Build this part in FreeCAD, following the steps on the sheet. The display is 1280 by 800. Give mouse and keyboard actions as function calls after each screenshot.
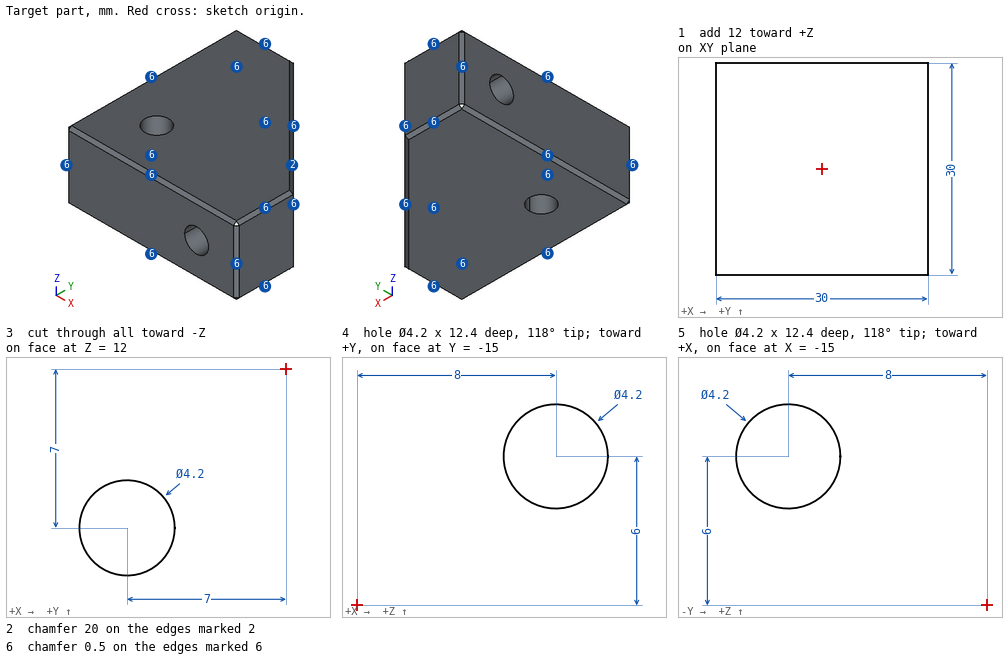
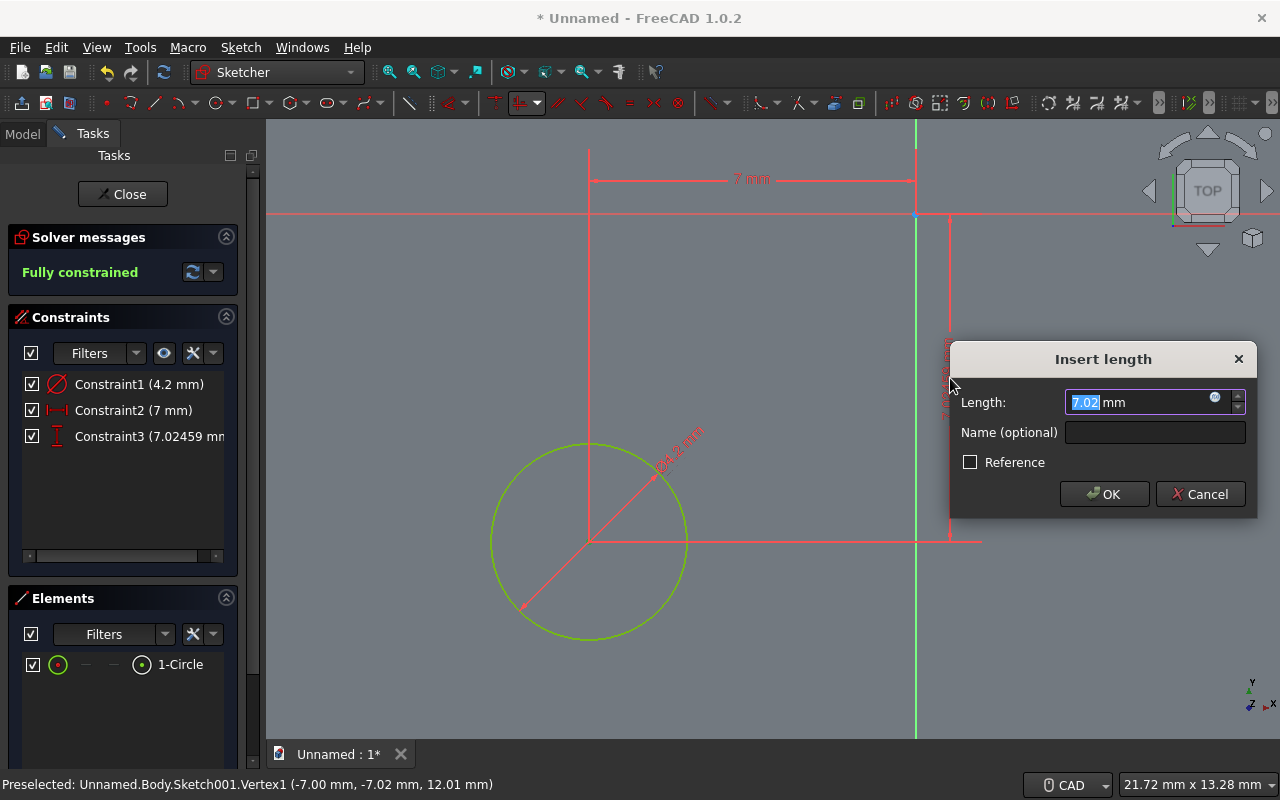
text(7)
key(Return)
key(Escape)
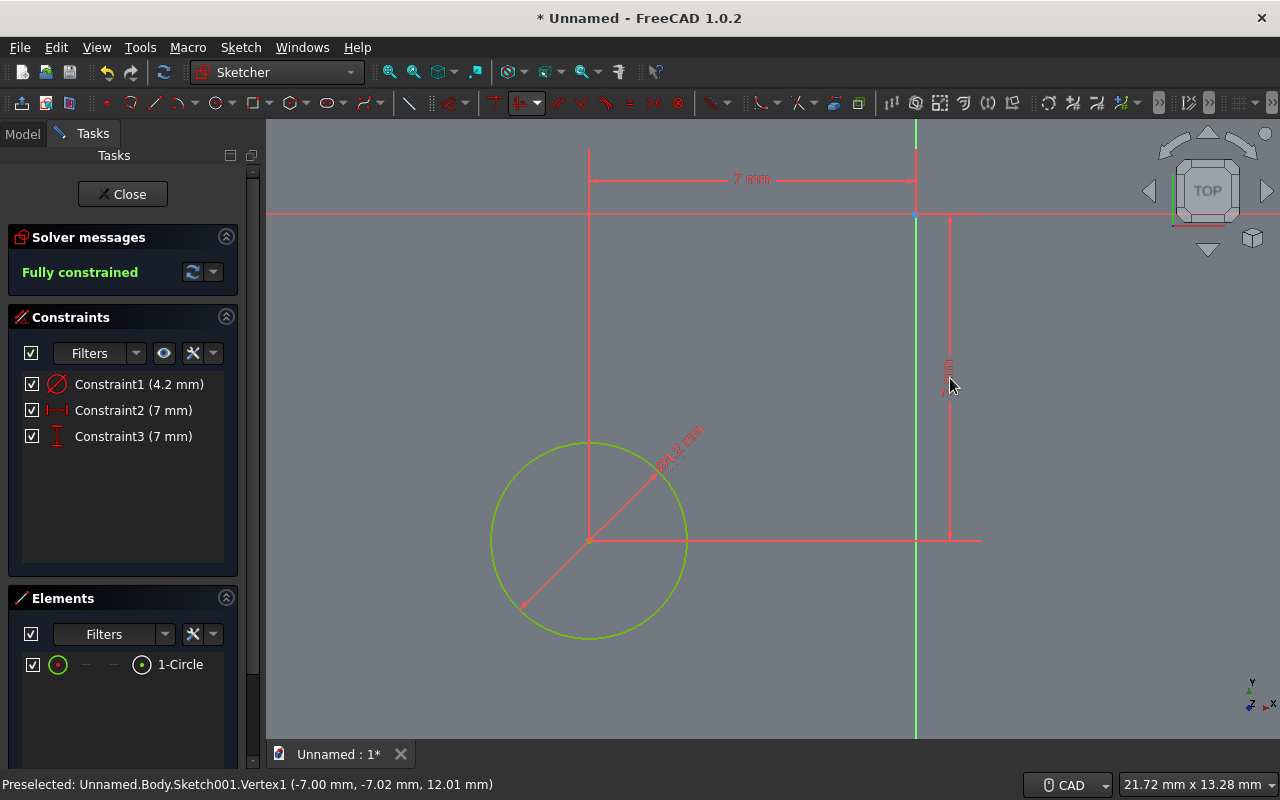
click(123, 194)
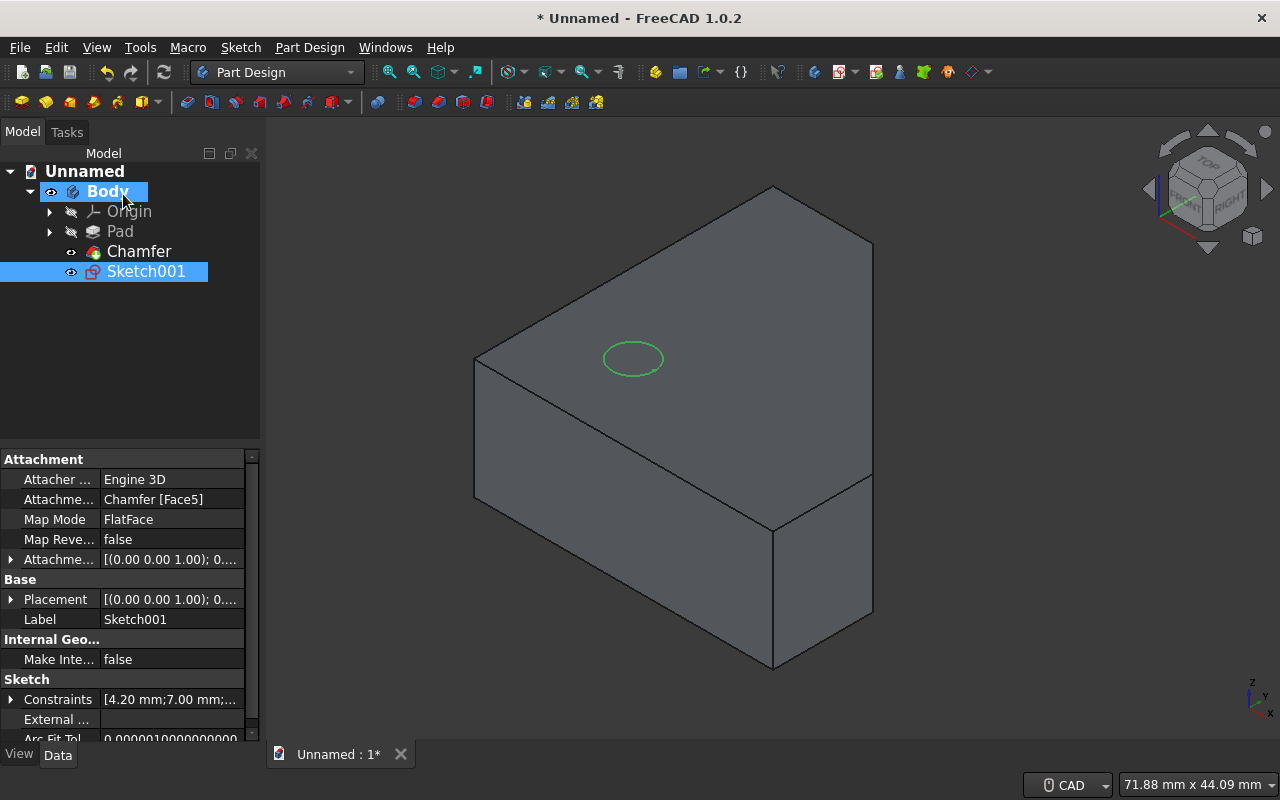
click(188, 102)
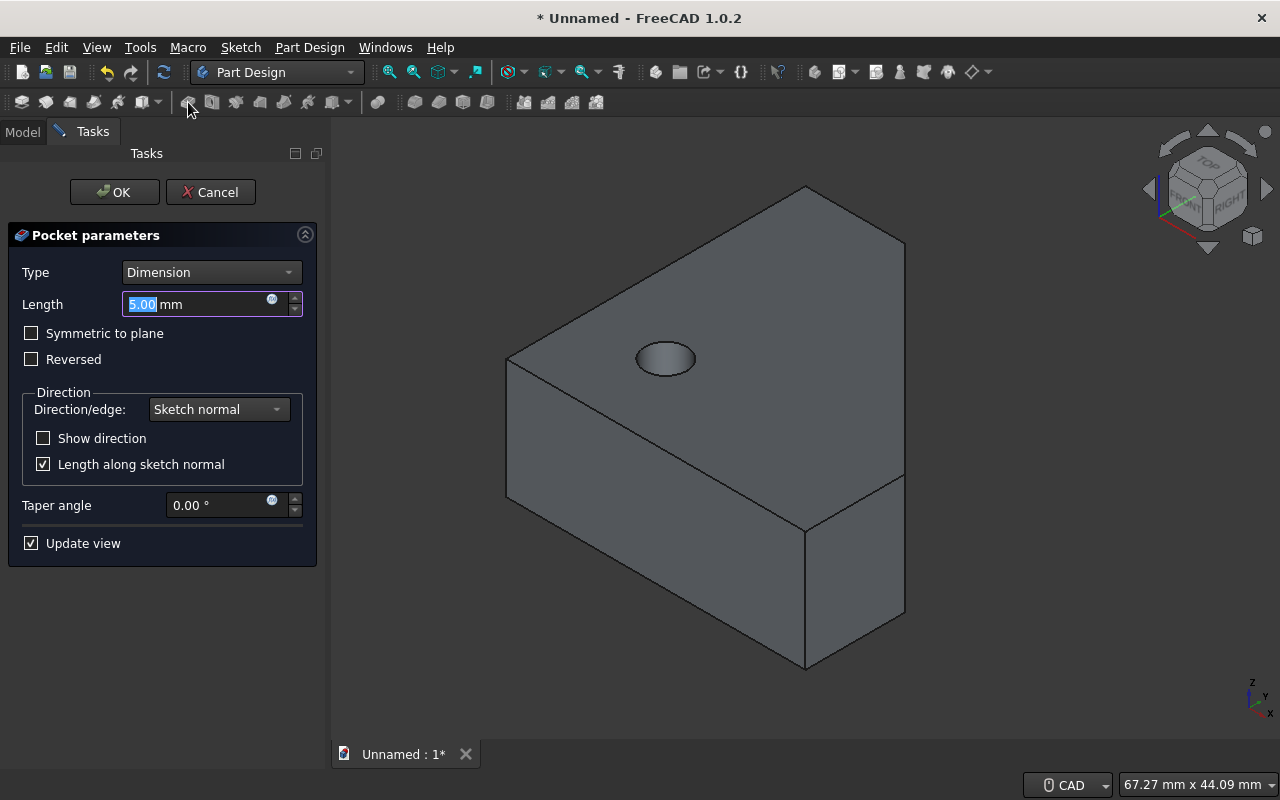
click(212, 272)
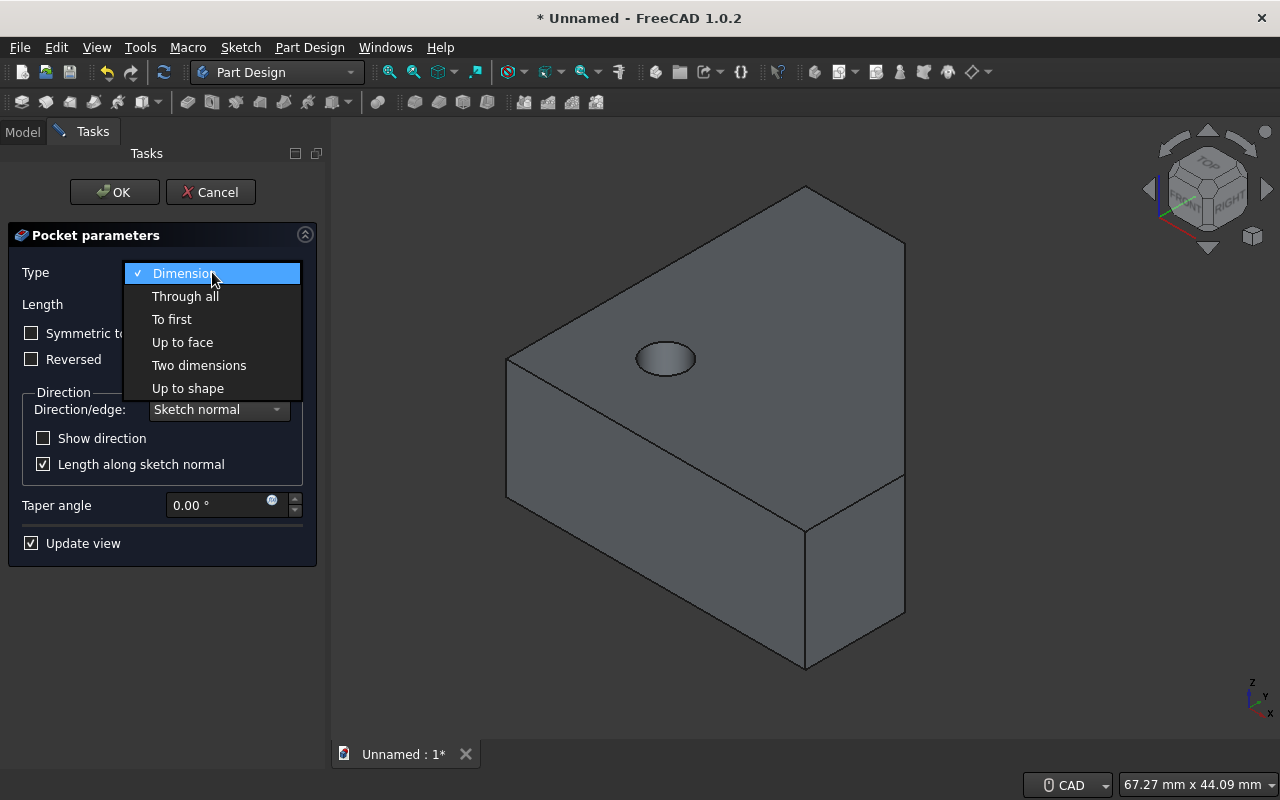
click(212, 296)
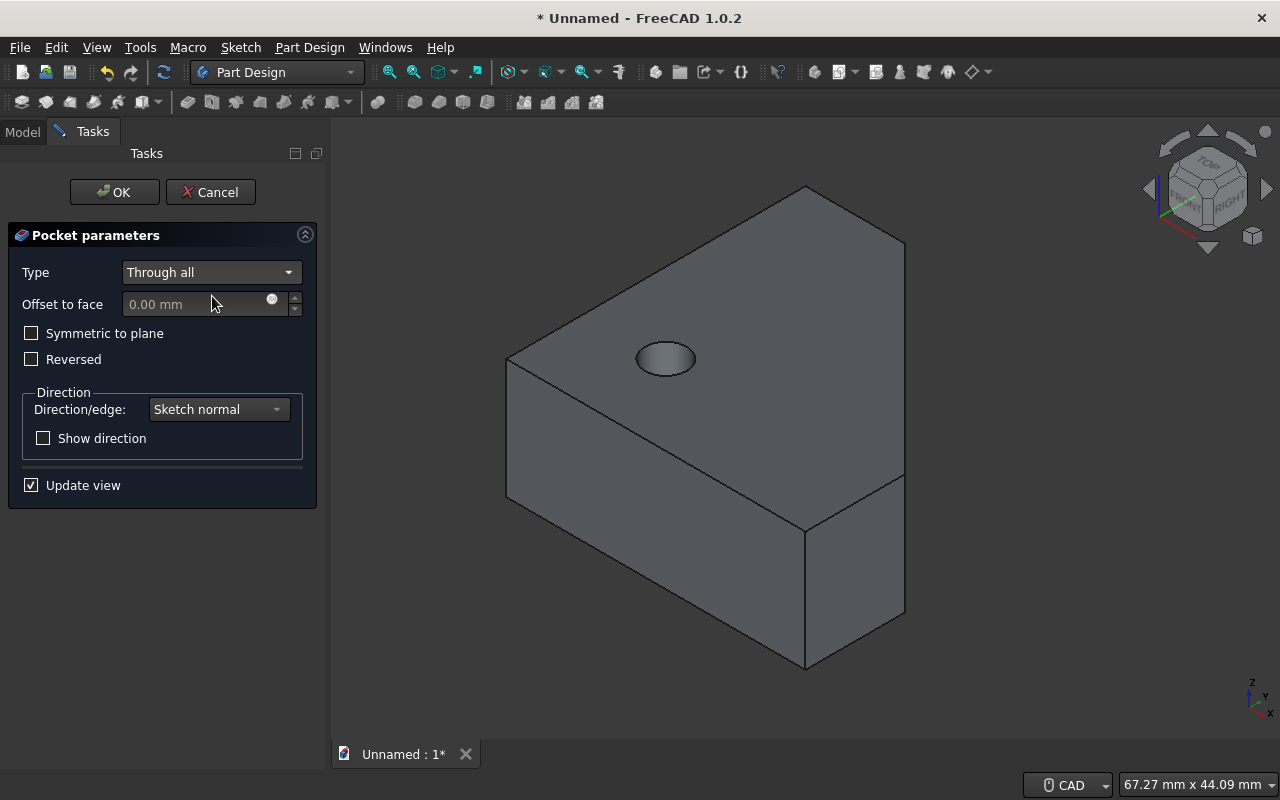
click(115, 192)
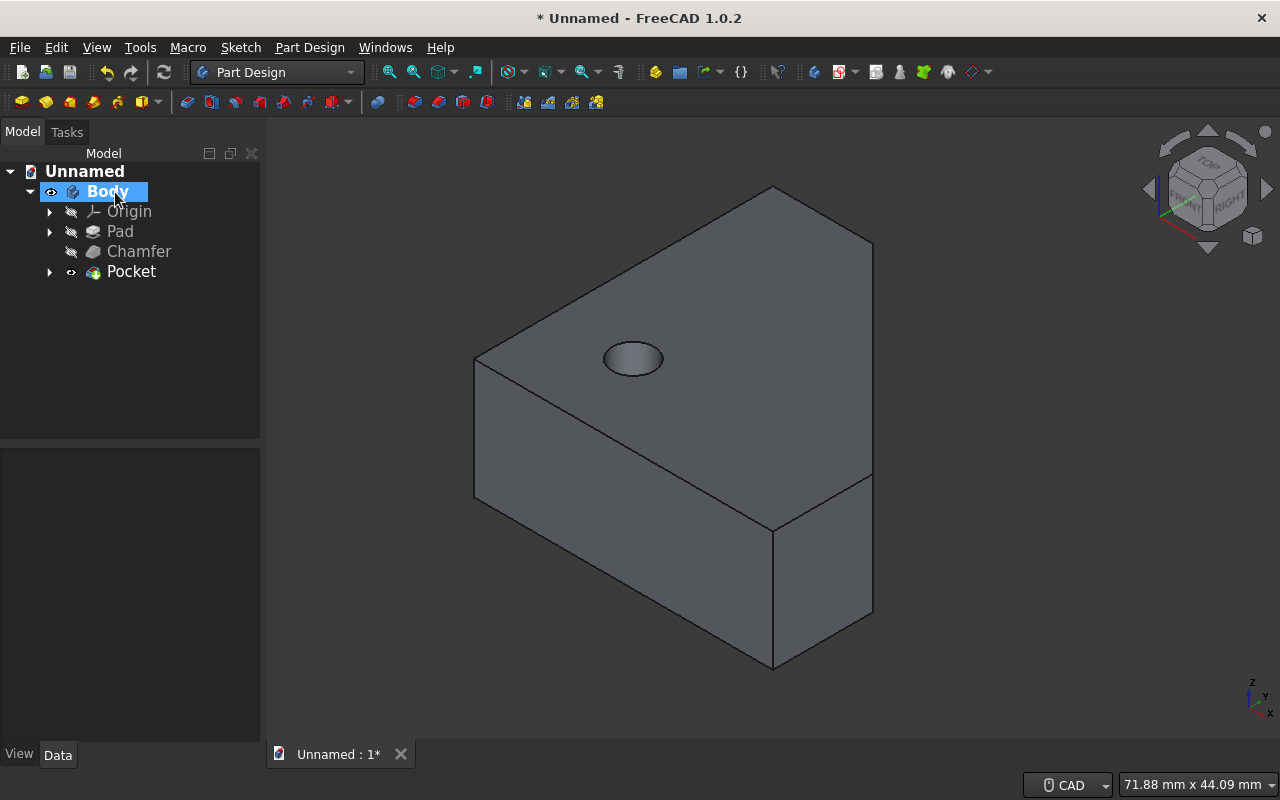
click(709, 563)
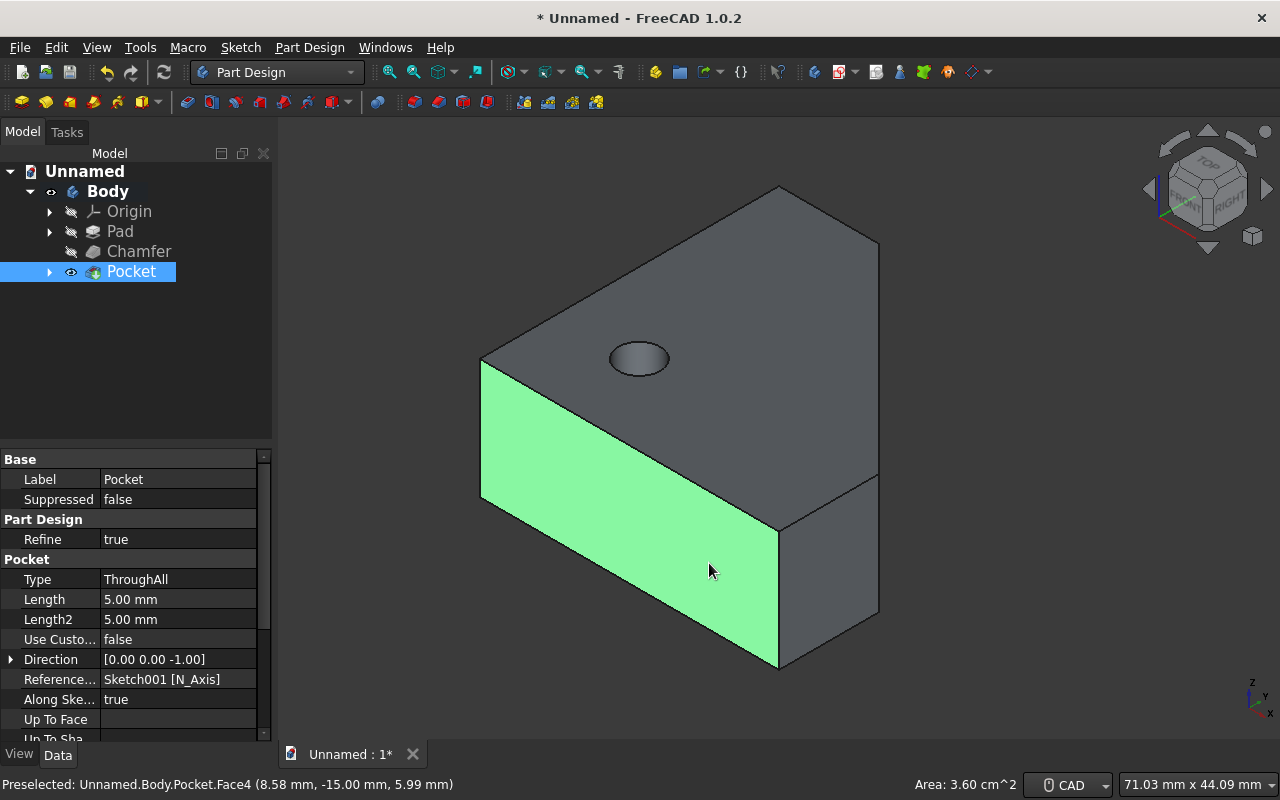
click(840, 72)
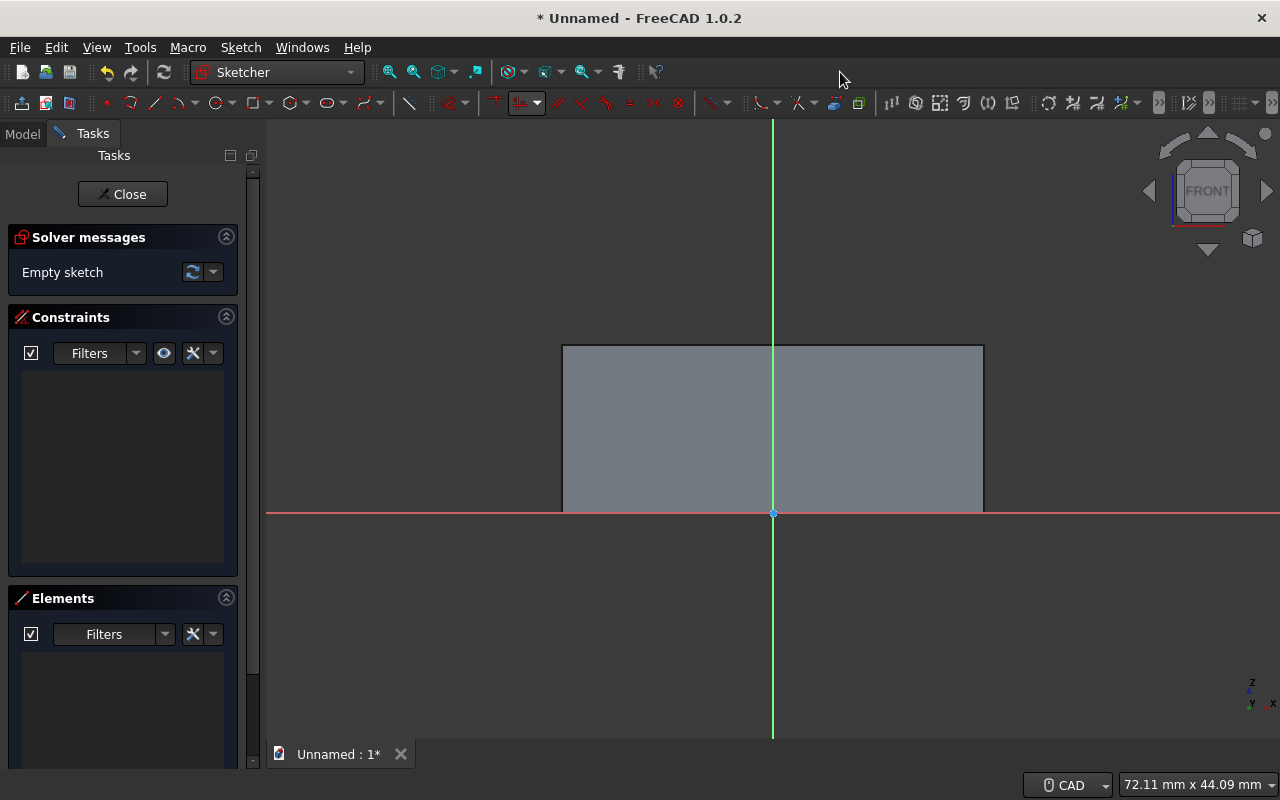
scroll(904, 468, up, 6)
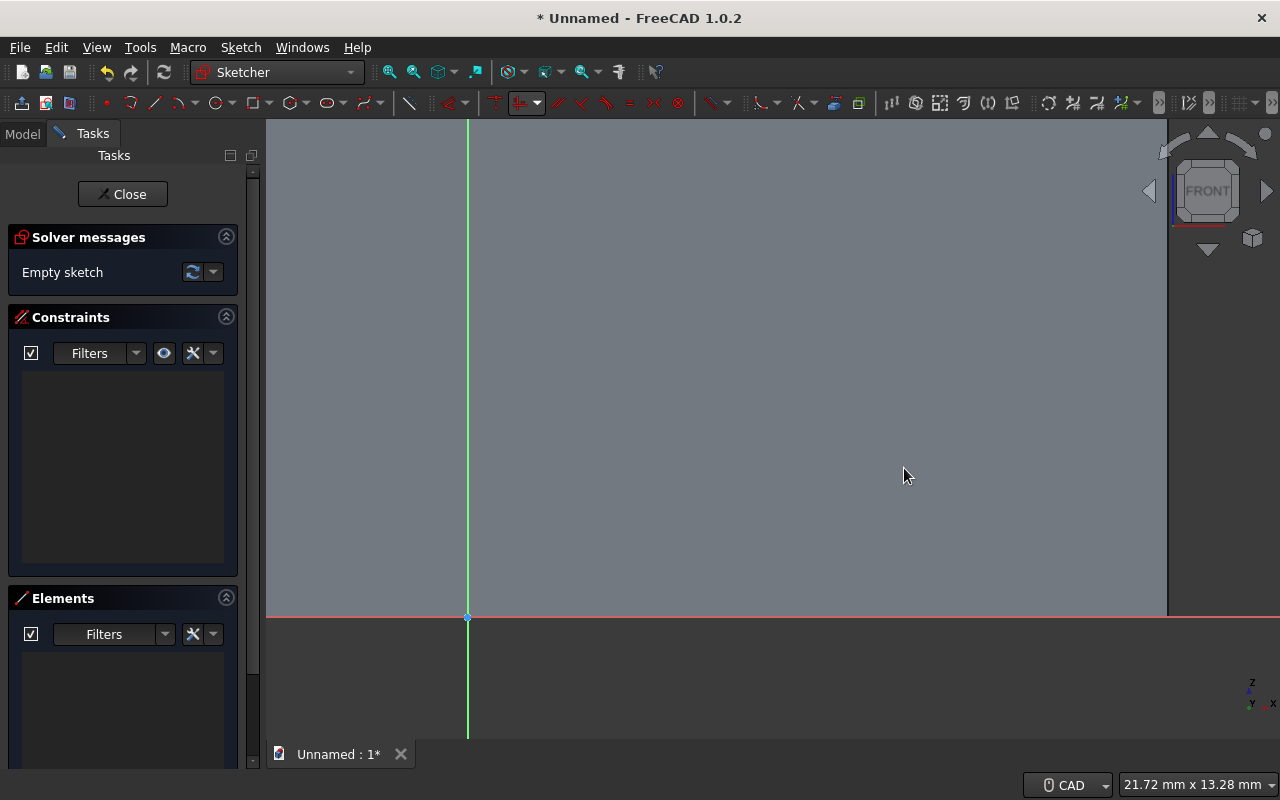
key(g)
key(c)